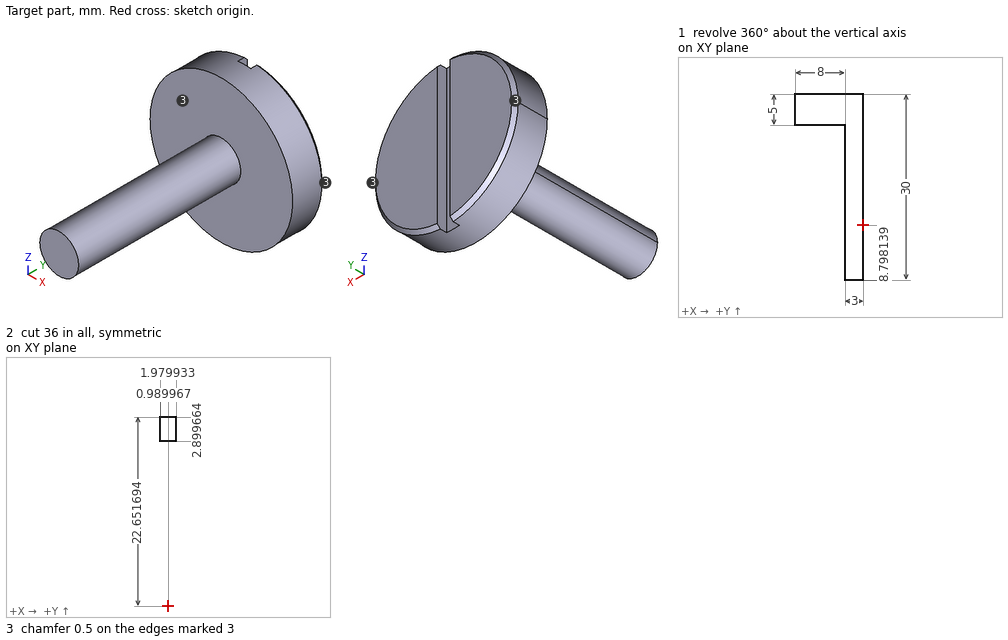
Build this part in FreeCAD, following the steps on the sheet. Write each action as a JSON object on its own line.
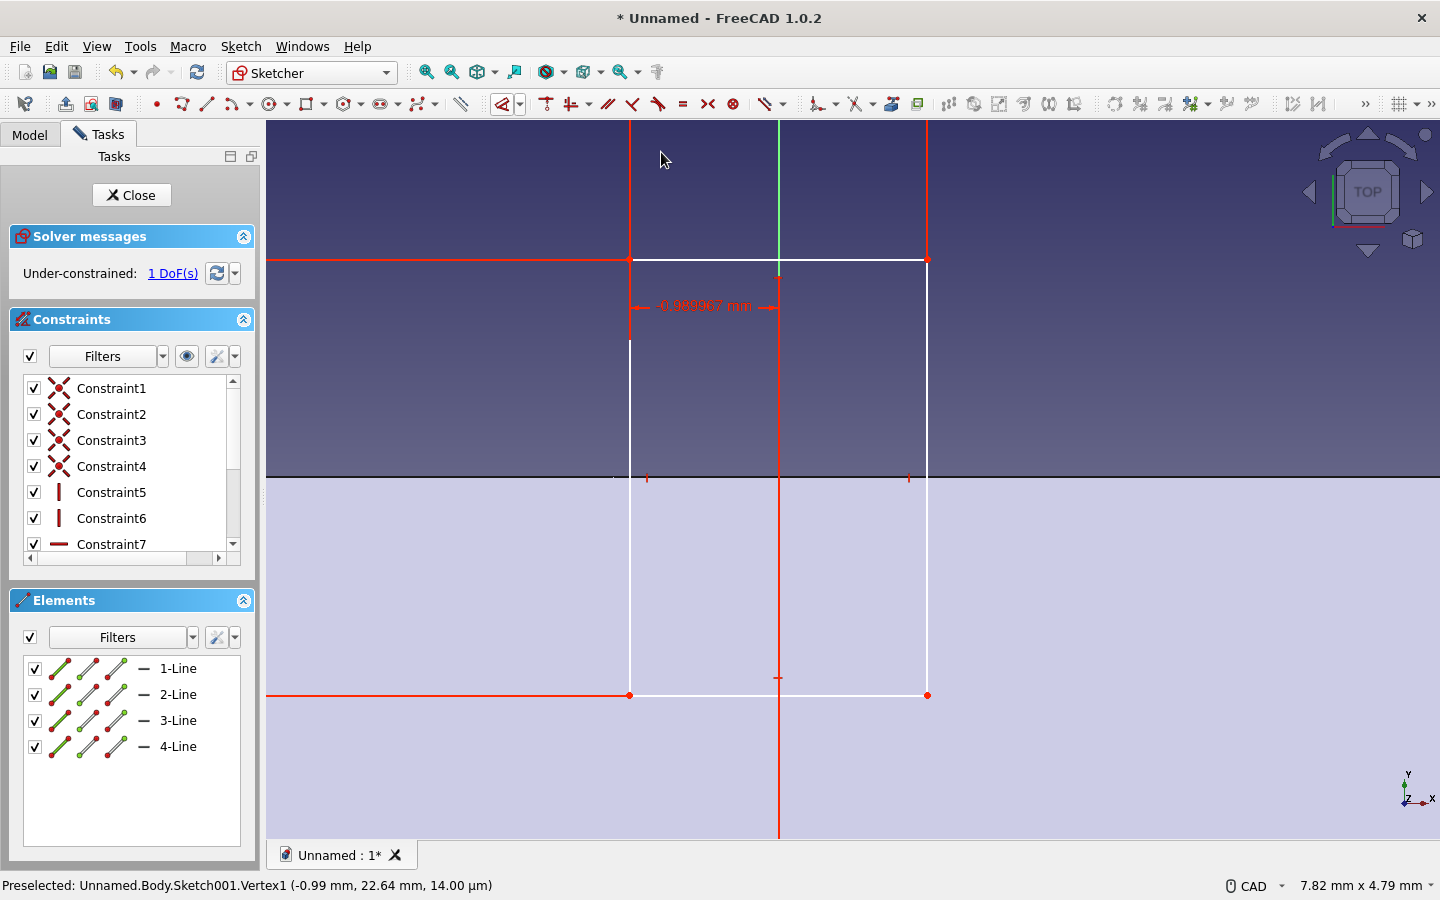
{"action": "left_click", "coordinate": [630, 260]}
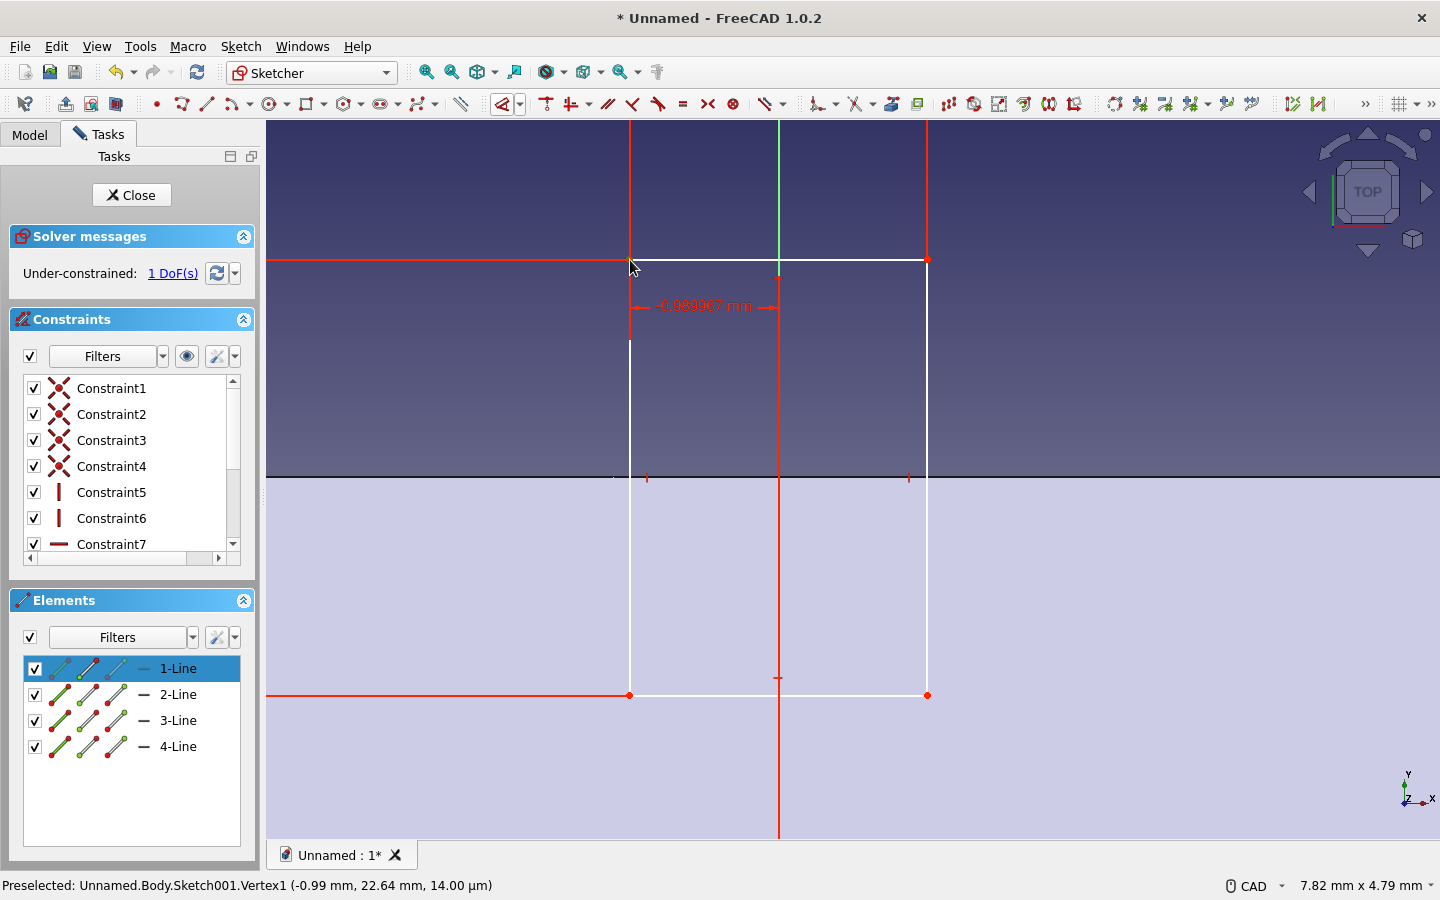
{"action": "key", "text": "i"}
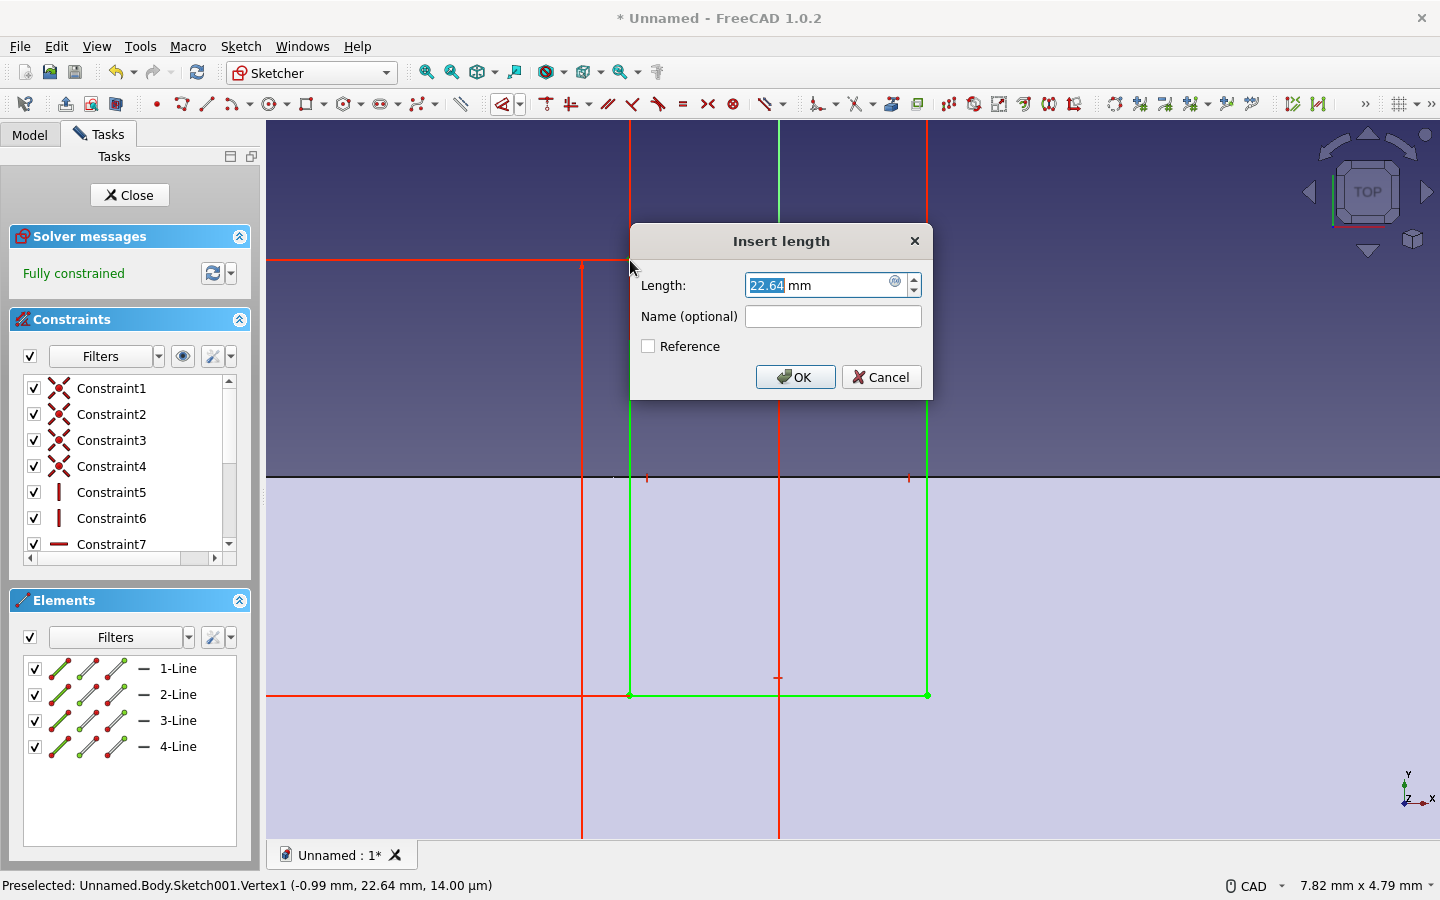
{"action": "type", "text": "22.651694"}
{"action": "key", "text": "Return"}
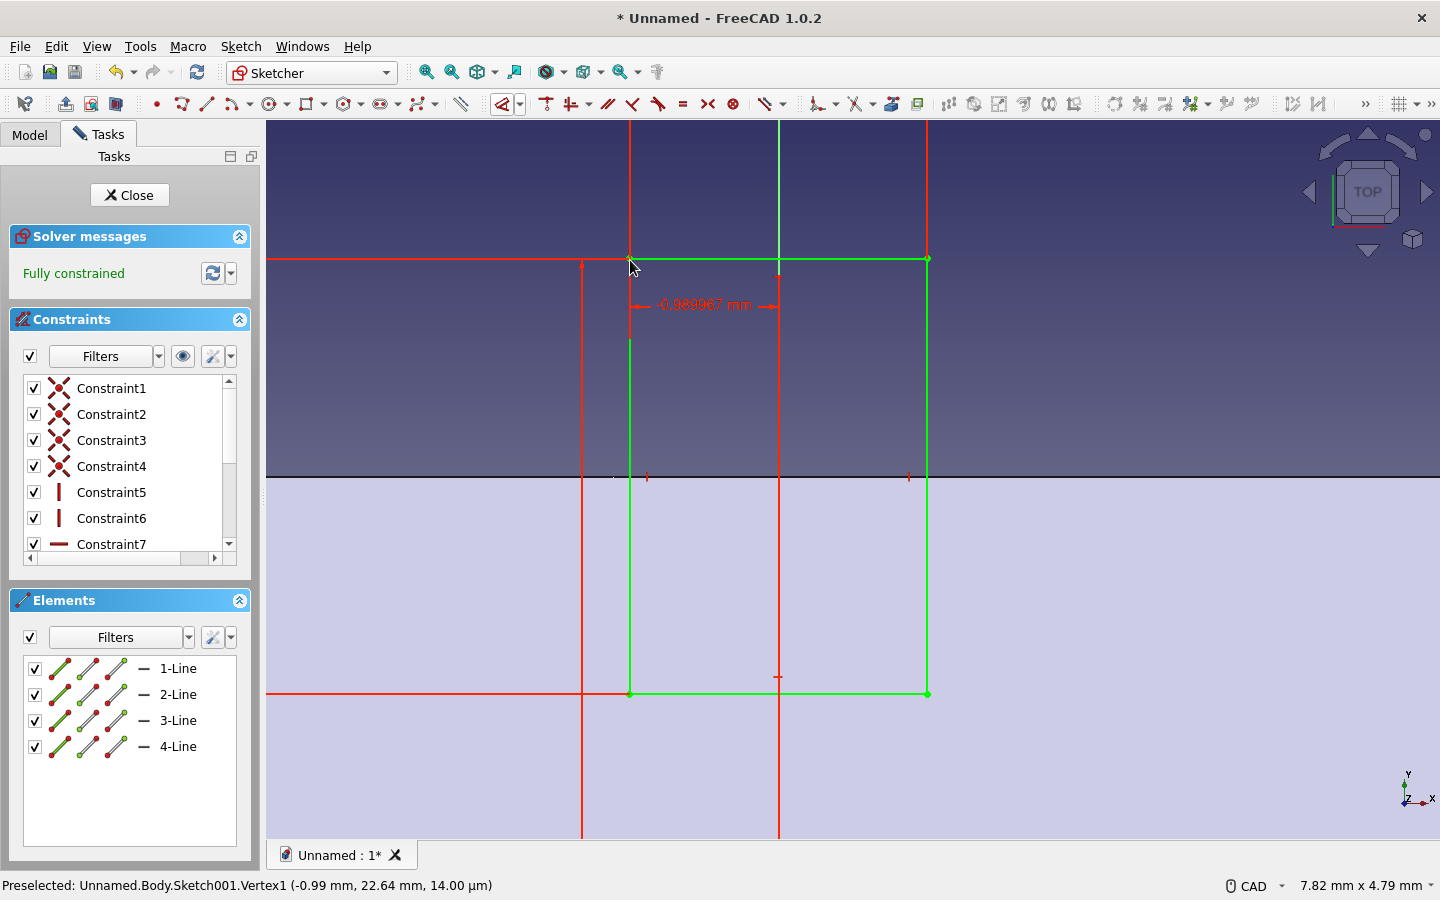
{"action": "left_click", "coordinate": [130, 195]}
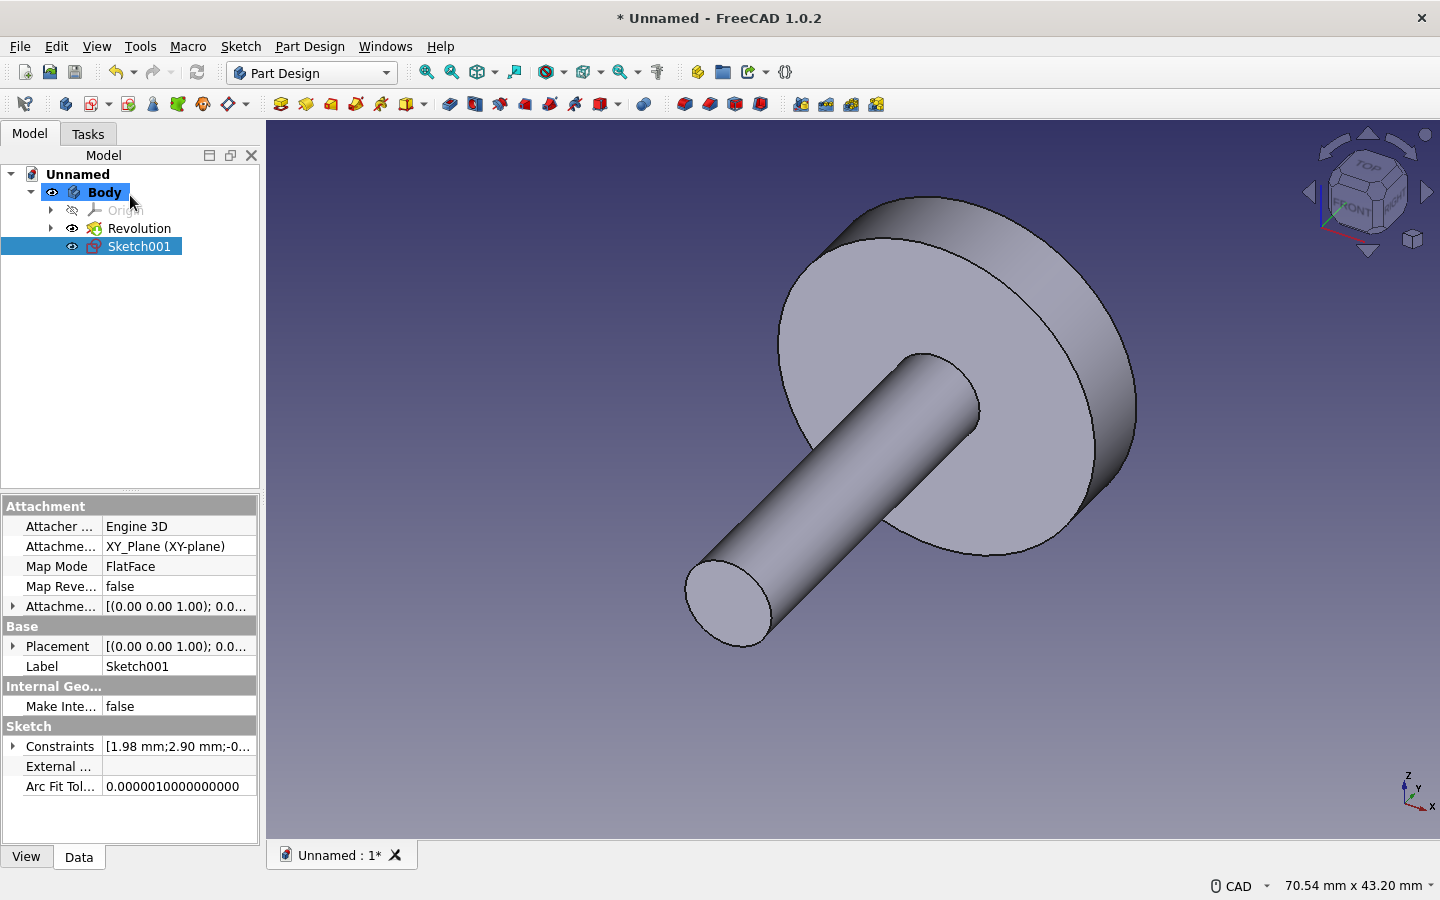
{"action": "left_click", "coordinate": [450, 104]}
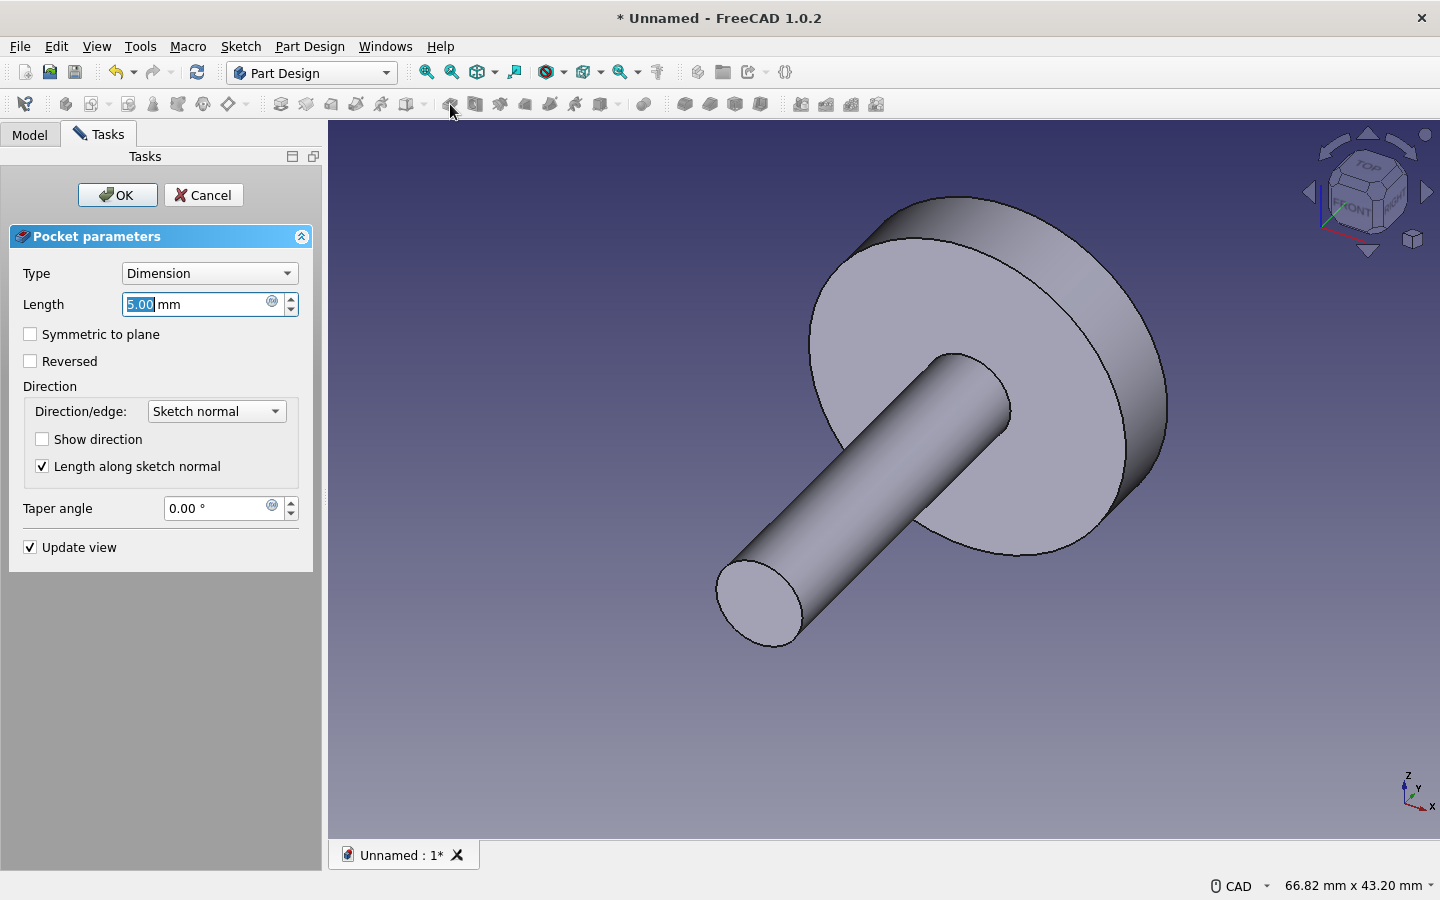
{"action": "type", "text": "36"}
{"action": "key", "text": "Tab"}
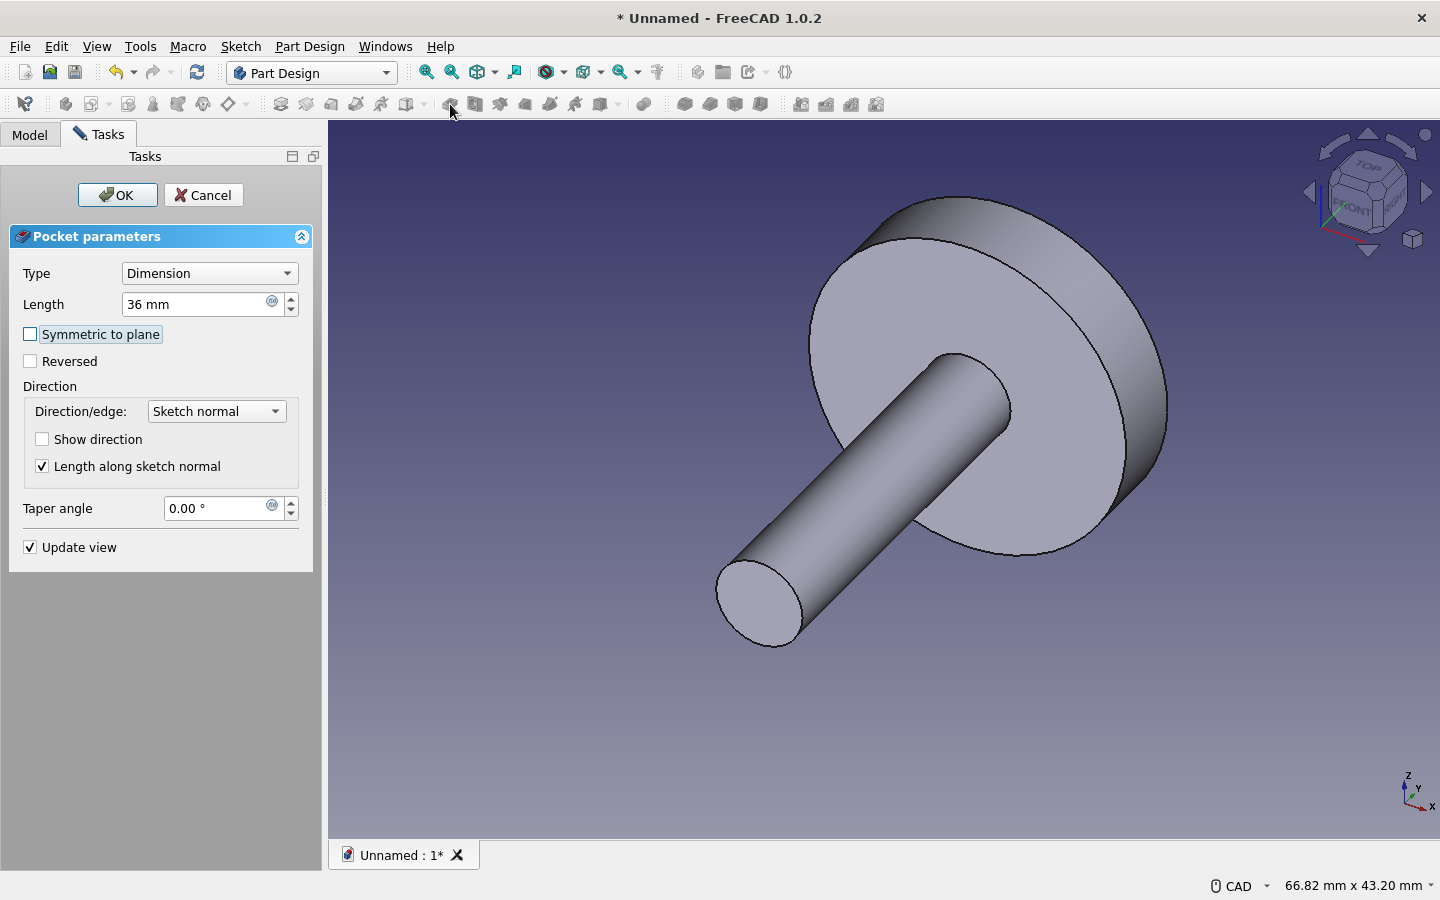
{"action": "left_click", "coordinate": [31, 334]}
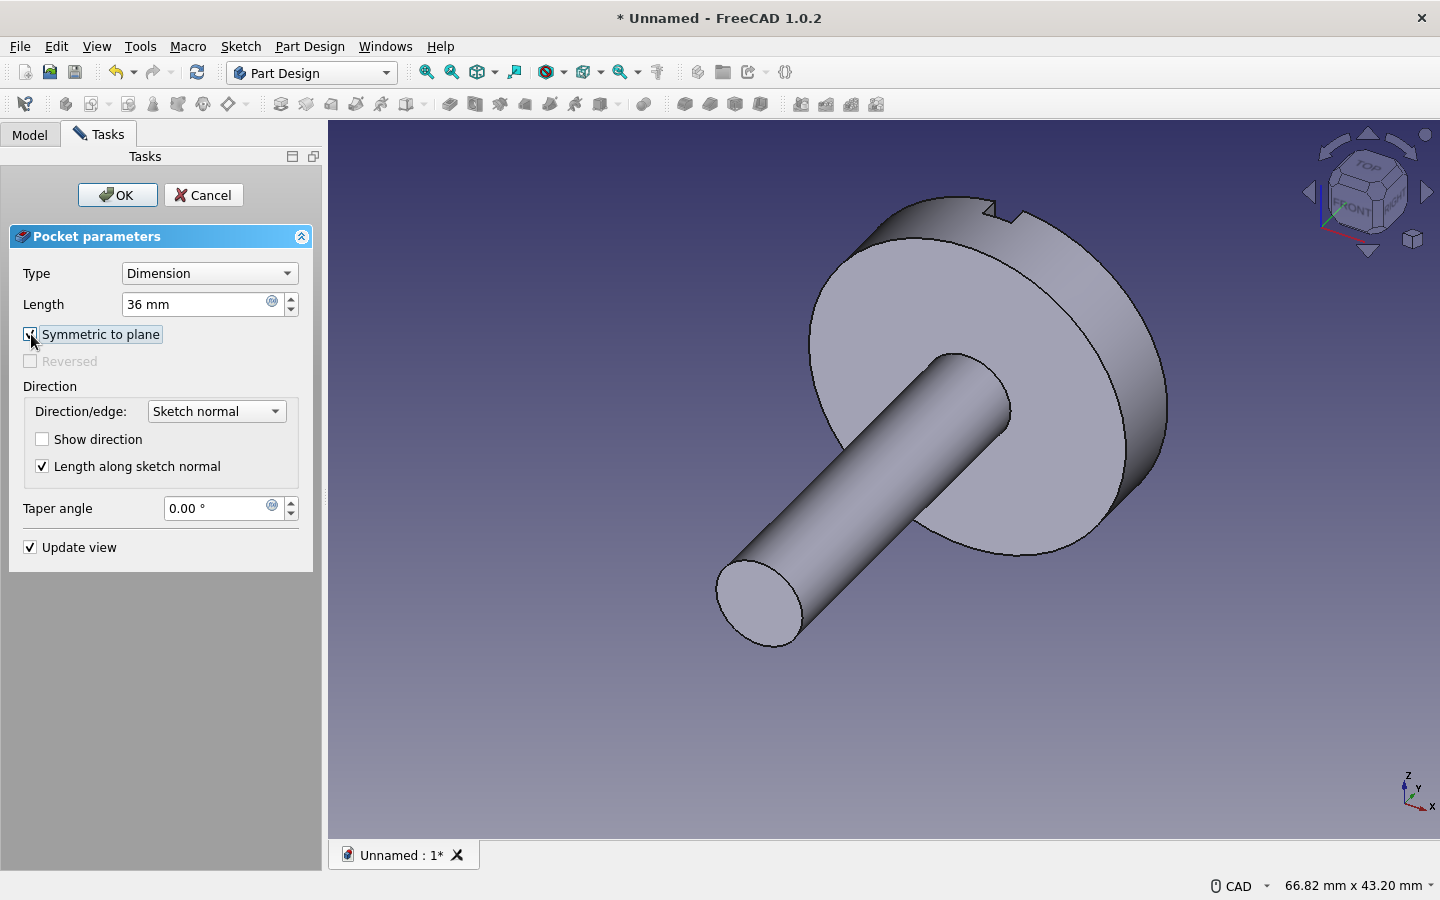
{"action": "left_click", "coordinate": [118, 195]}